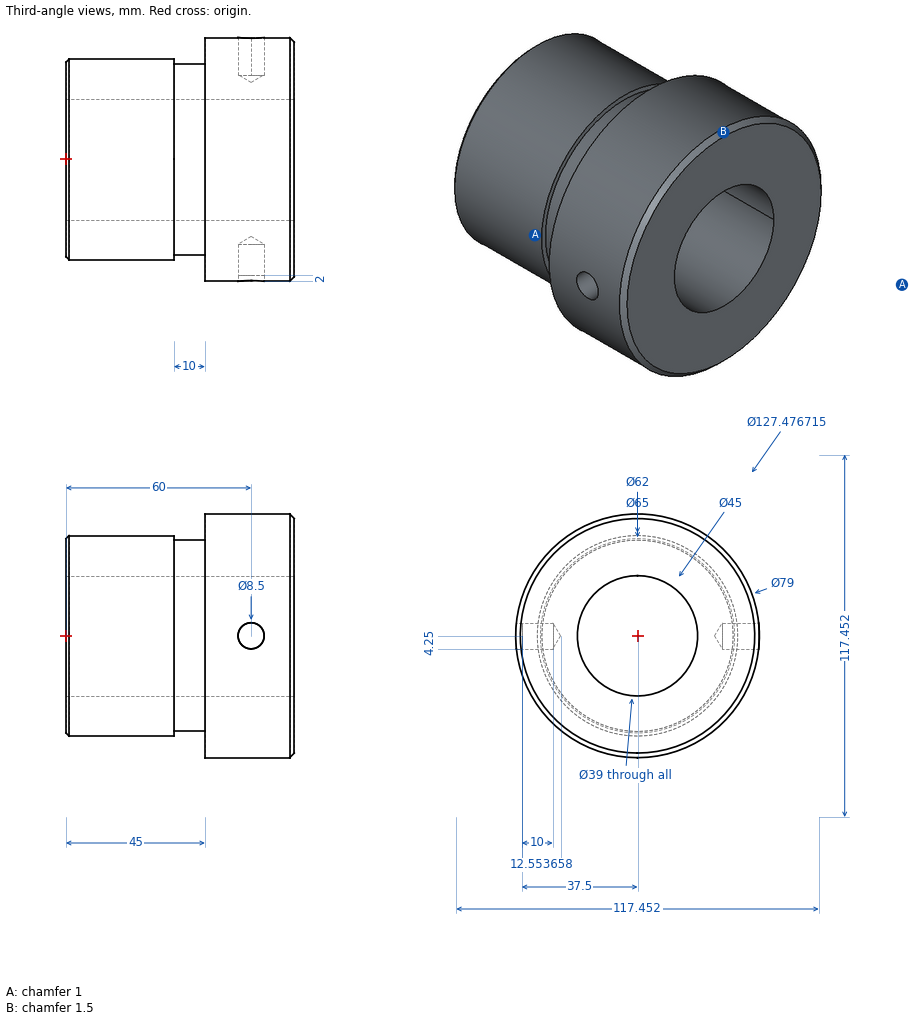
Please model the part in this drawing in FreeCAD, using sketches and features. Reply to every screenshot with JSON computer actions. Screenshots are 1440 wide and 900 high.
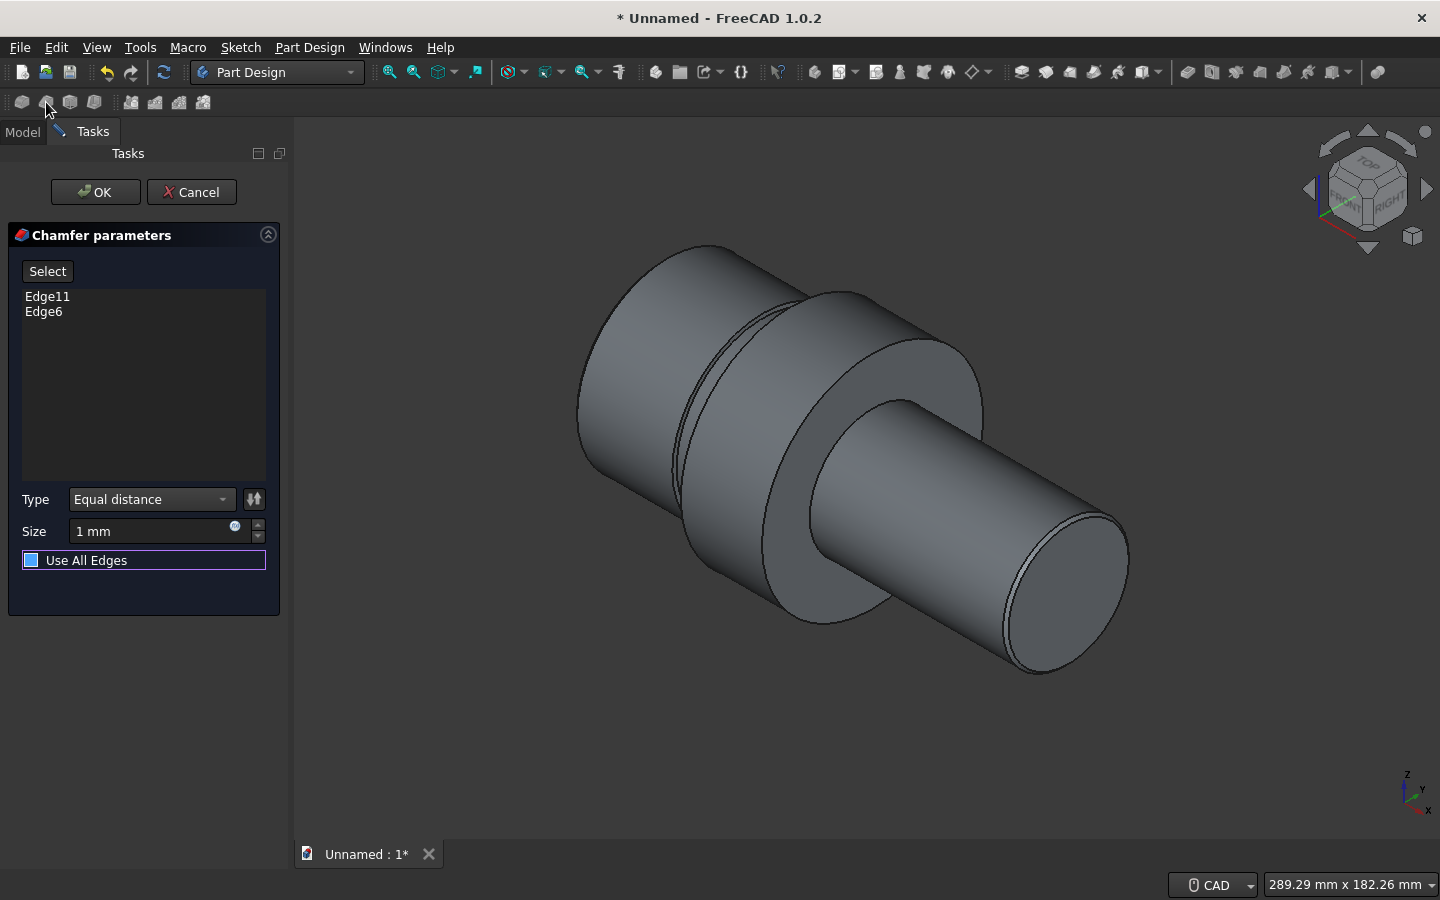
{"action": "left_click", "coordinate": [96, 192]}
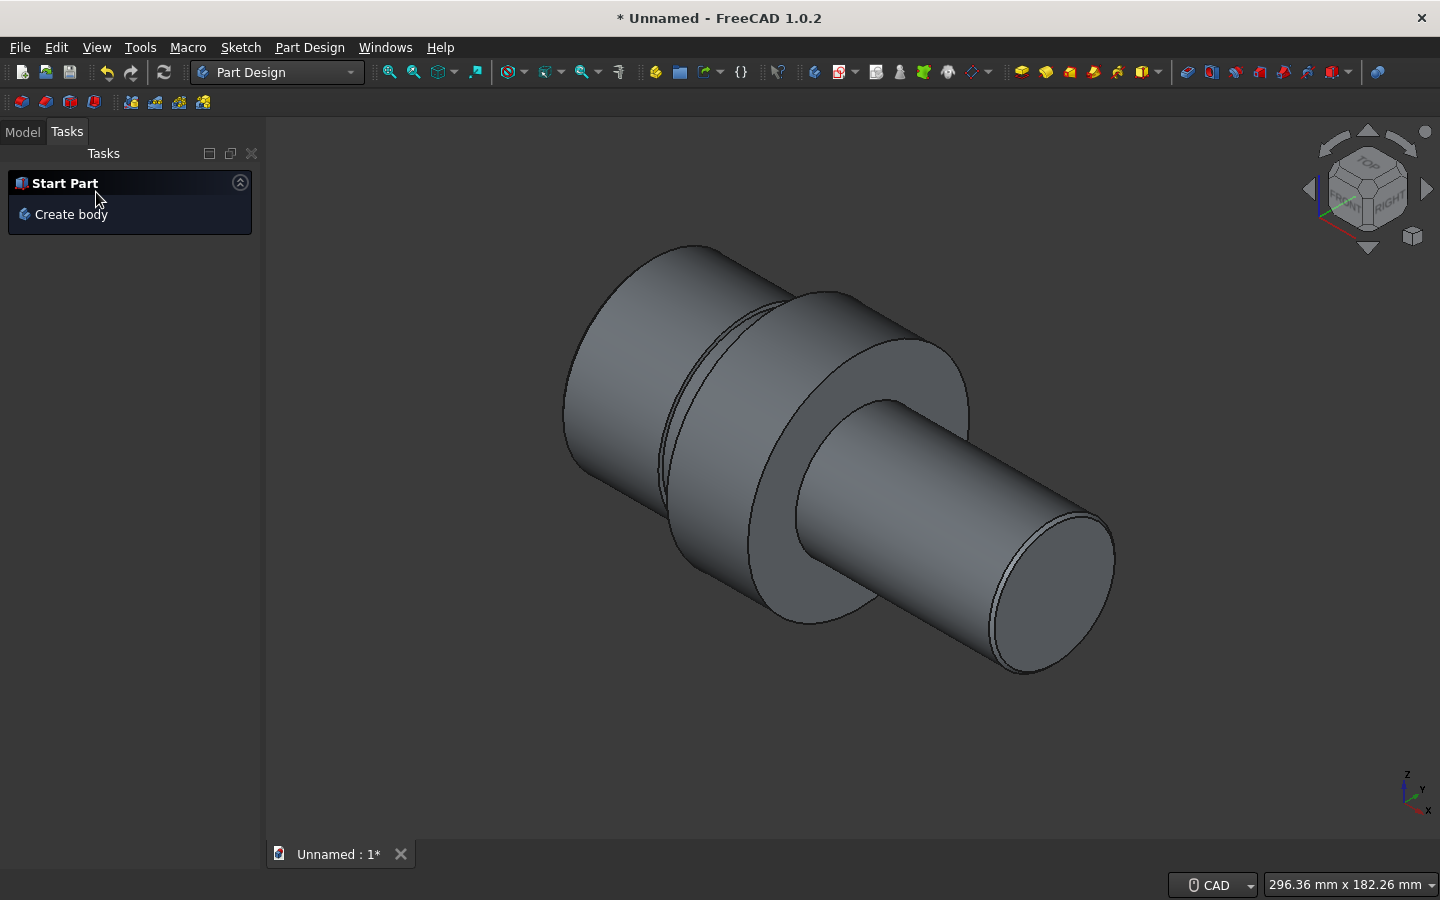
{"action": "left_click", "coordinate": [748, 544]}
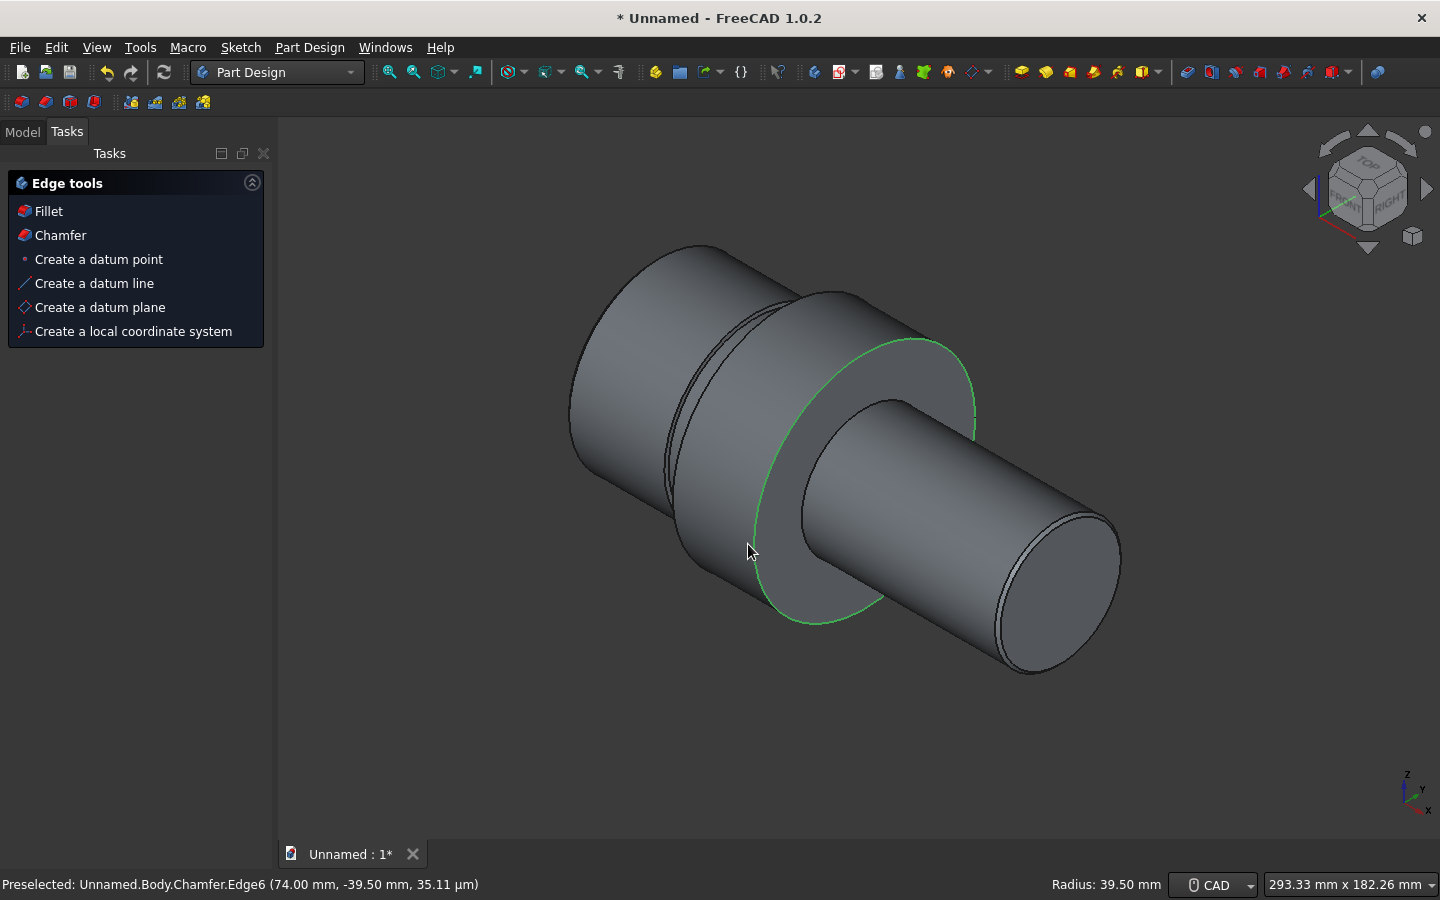
{"action": "left_click", "coordinate": [46, 102]}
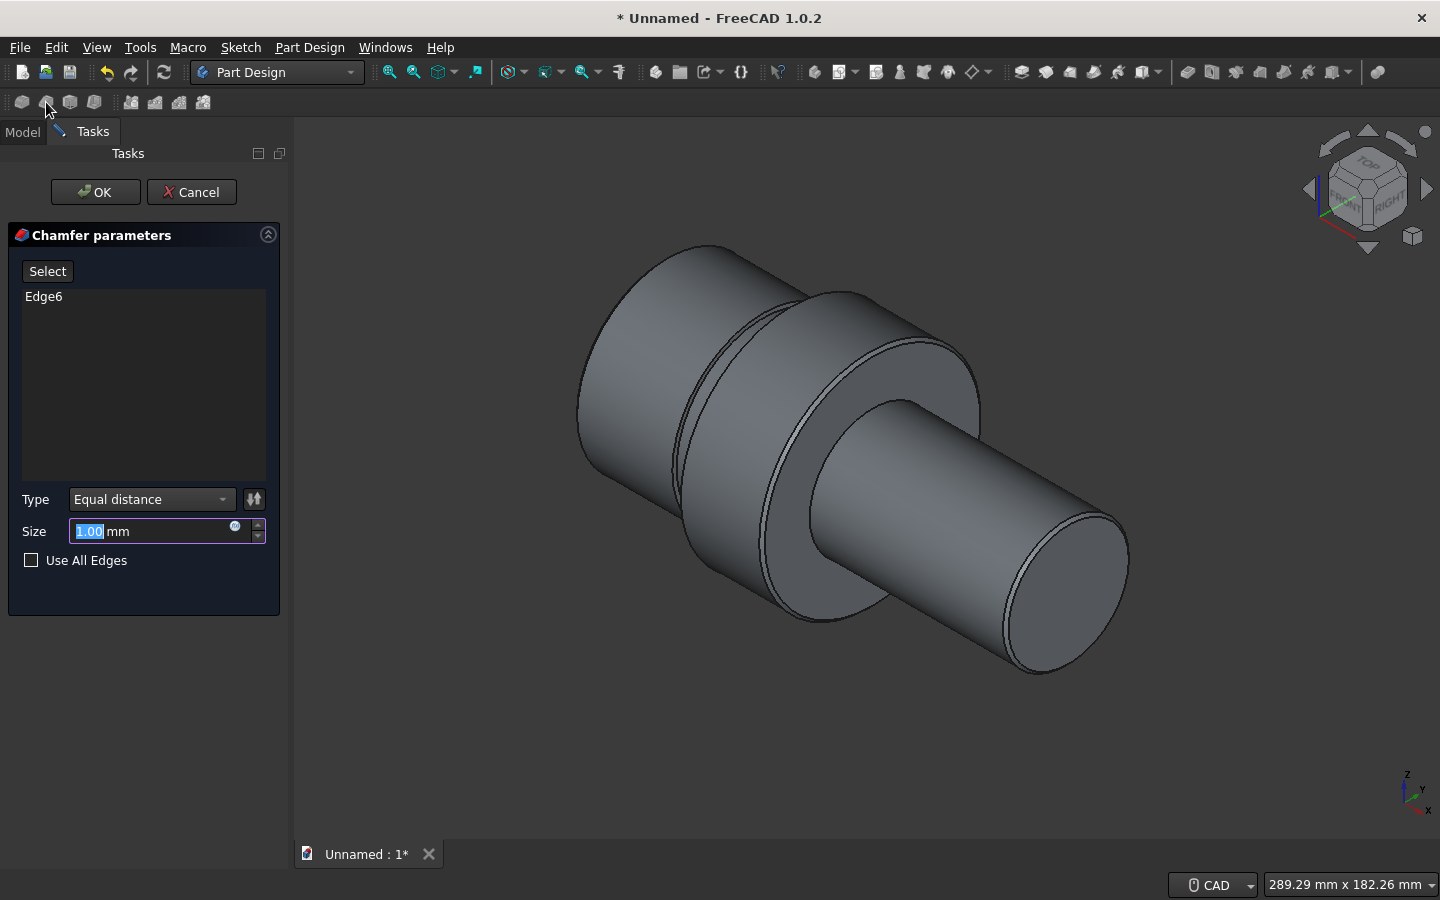
{"action": "type", "text": "1.5"}
{"action": "key", "text": "Tab"}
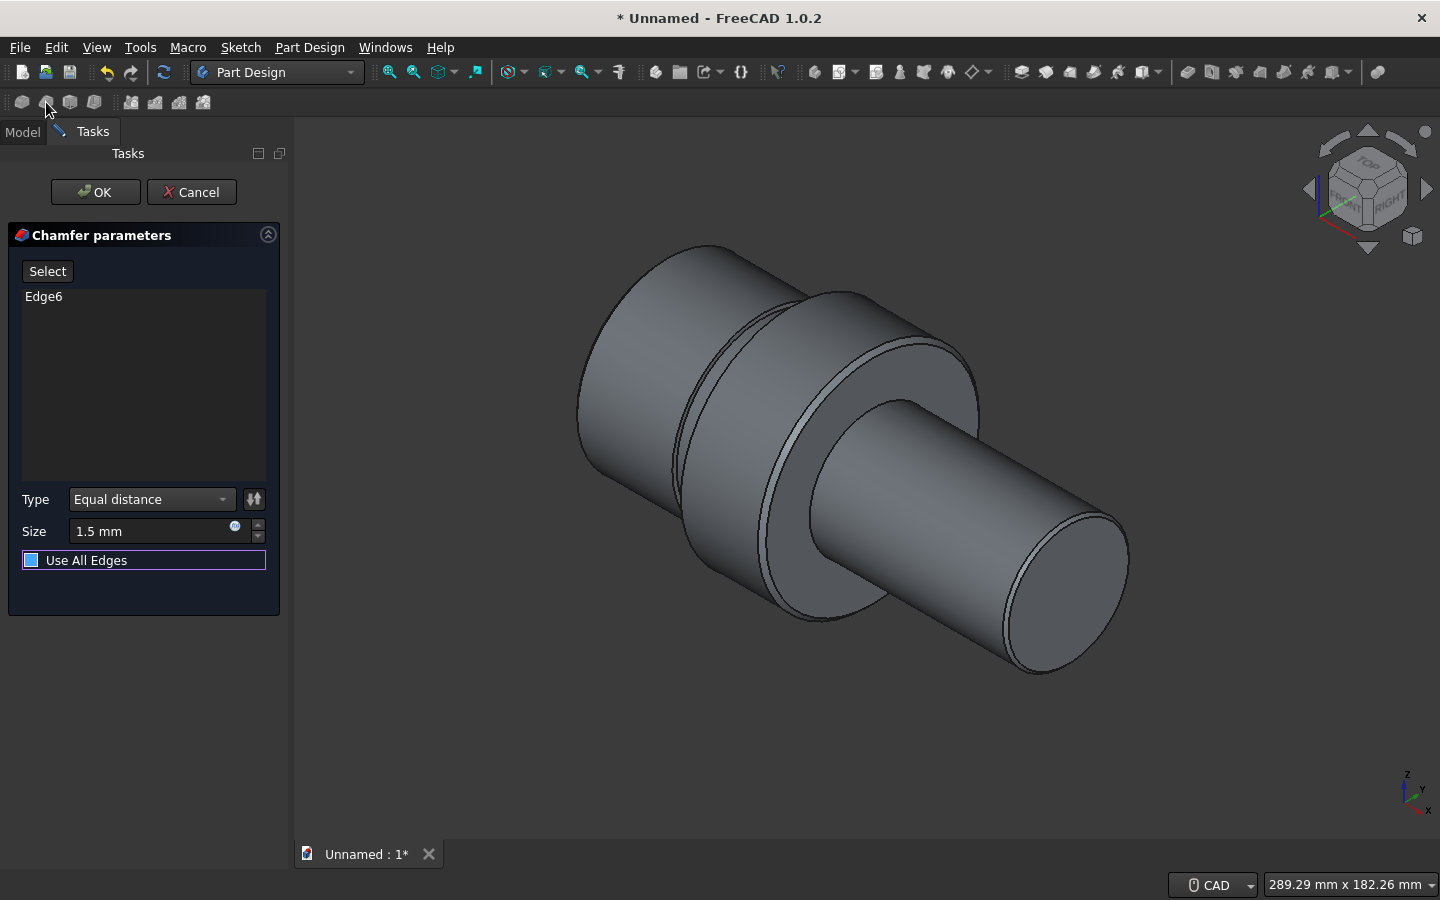
{"action": "left_click", "coordinate": [96, 192]}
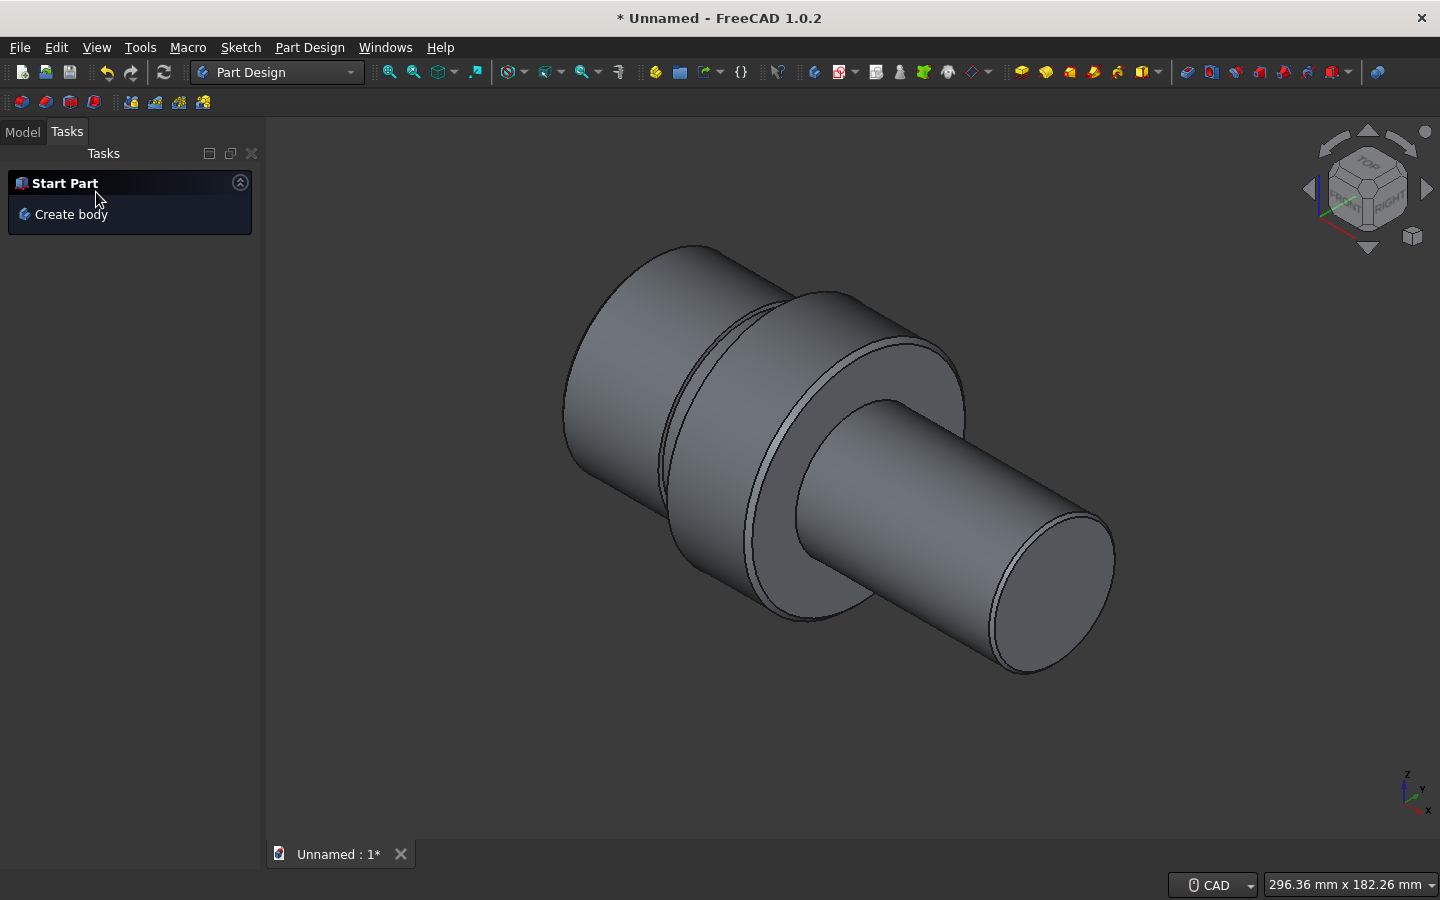
{"action": "left_click", "coordinate": [23, 131]}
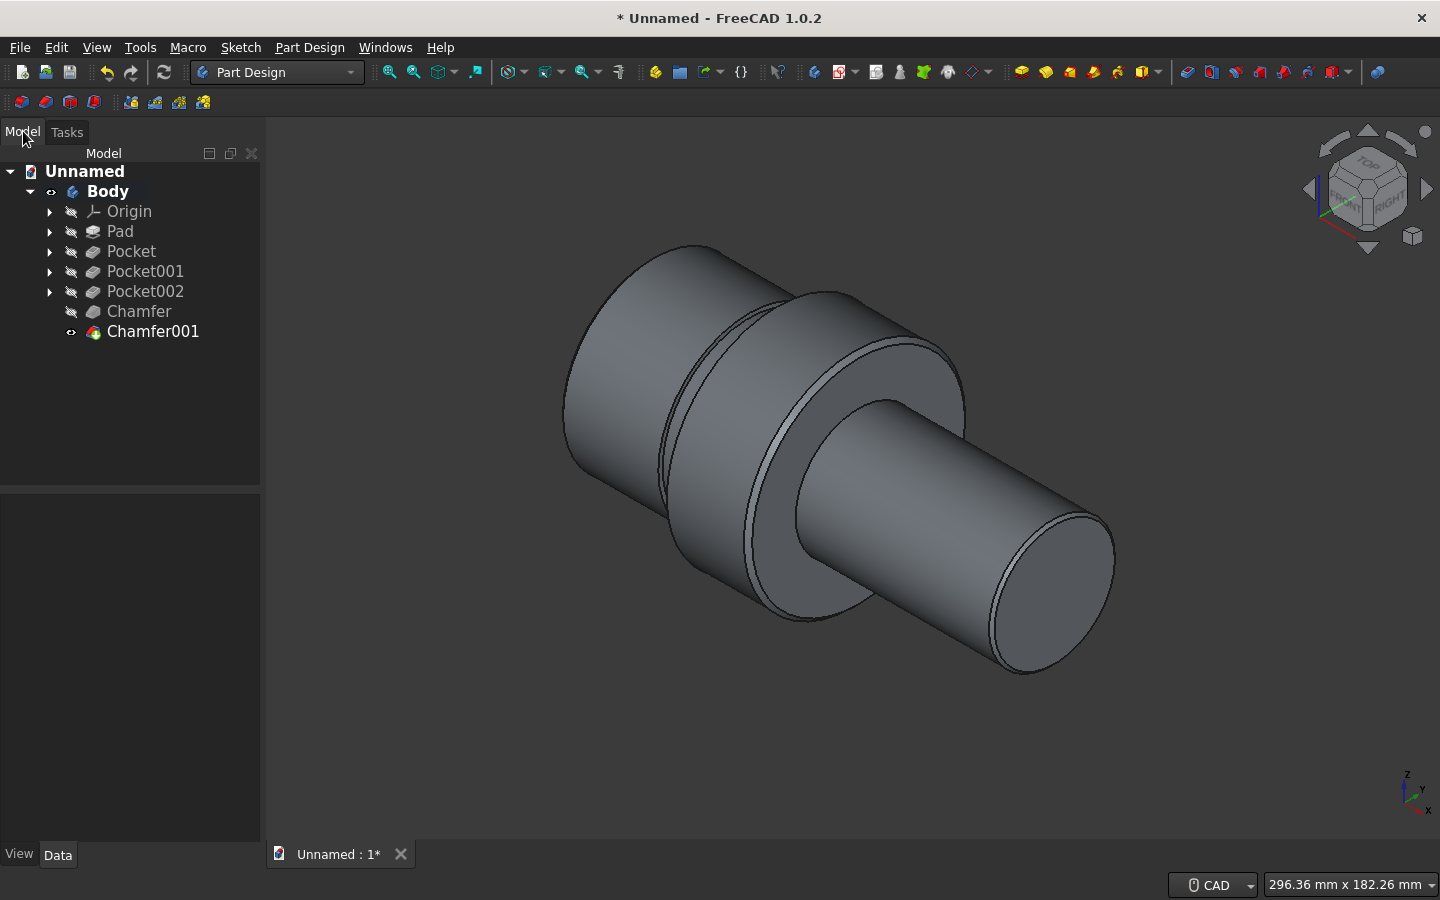
{"action": "left_click", "coordinate": [50, 212]}